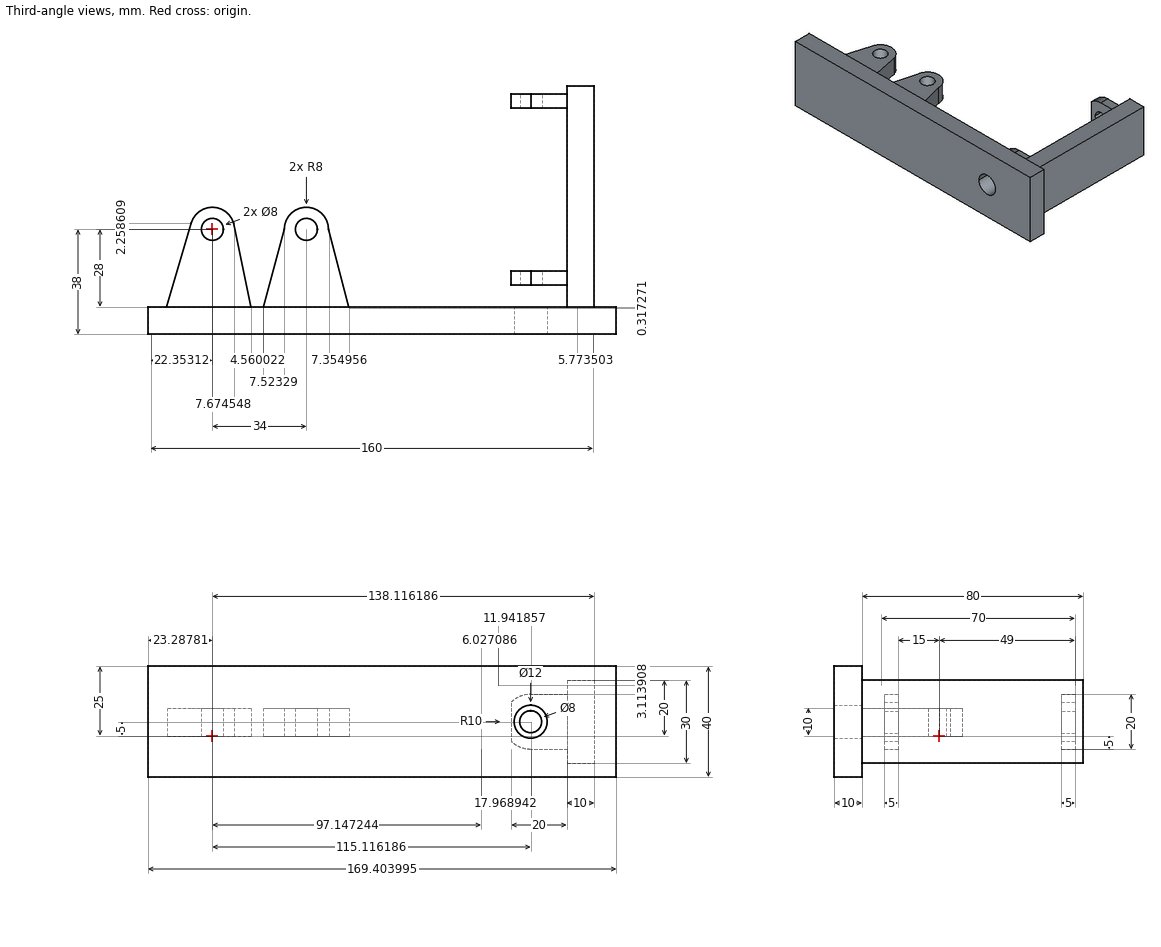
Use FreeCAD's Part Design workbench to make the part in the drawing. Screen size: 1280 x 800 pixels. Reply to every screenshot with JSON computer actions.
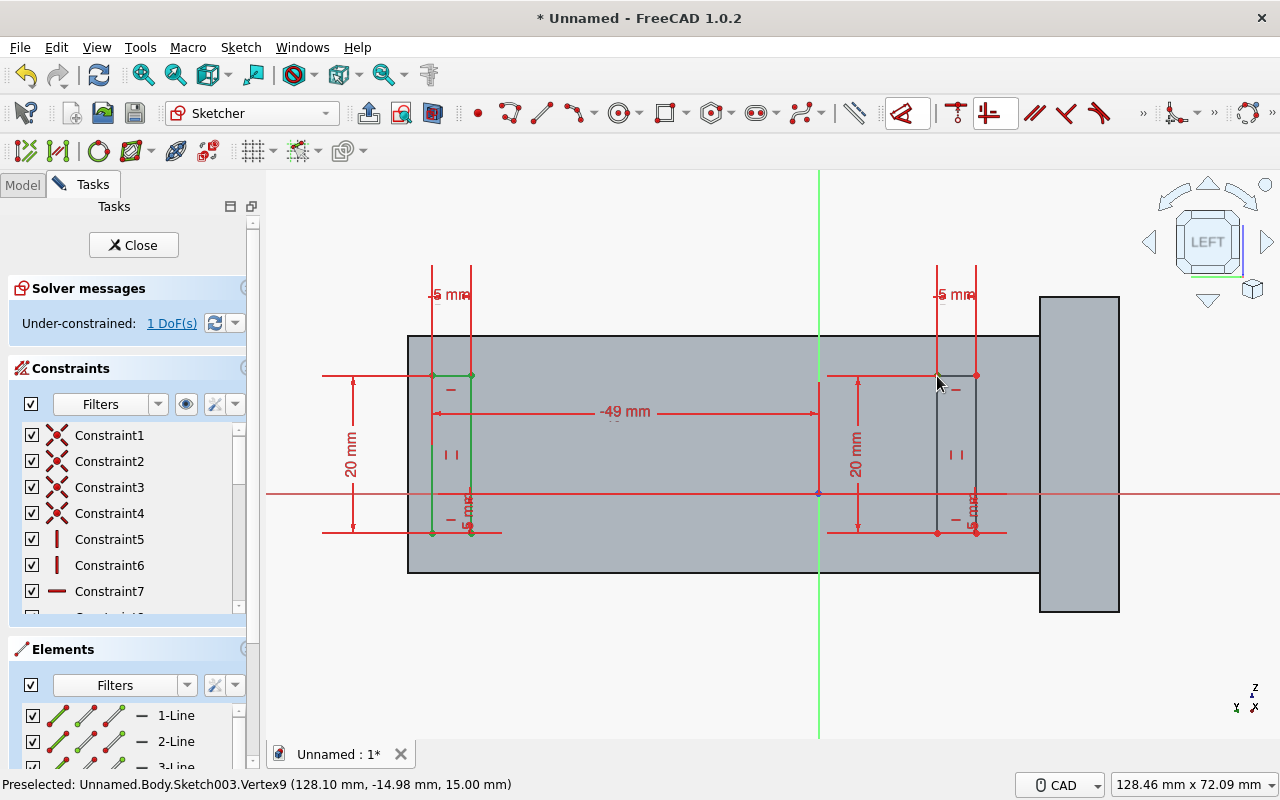
{"action": "key", "text": "l"}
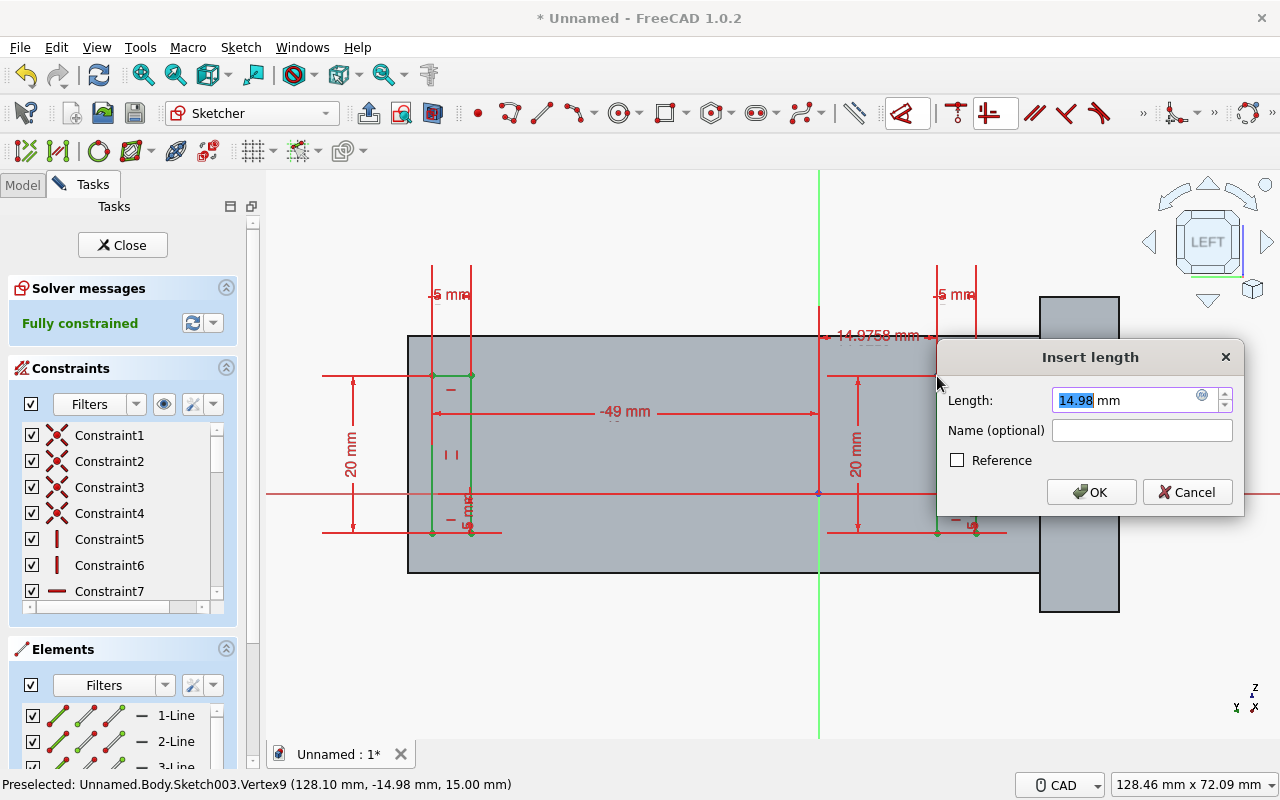
{"action": "type", "text": "15"}
{"action": "key", "text": "Return"}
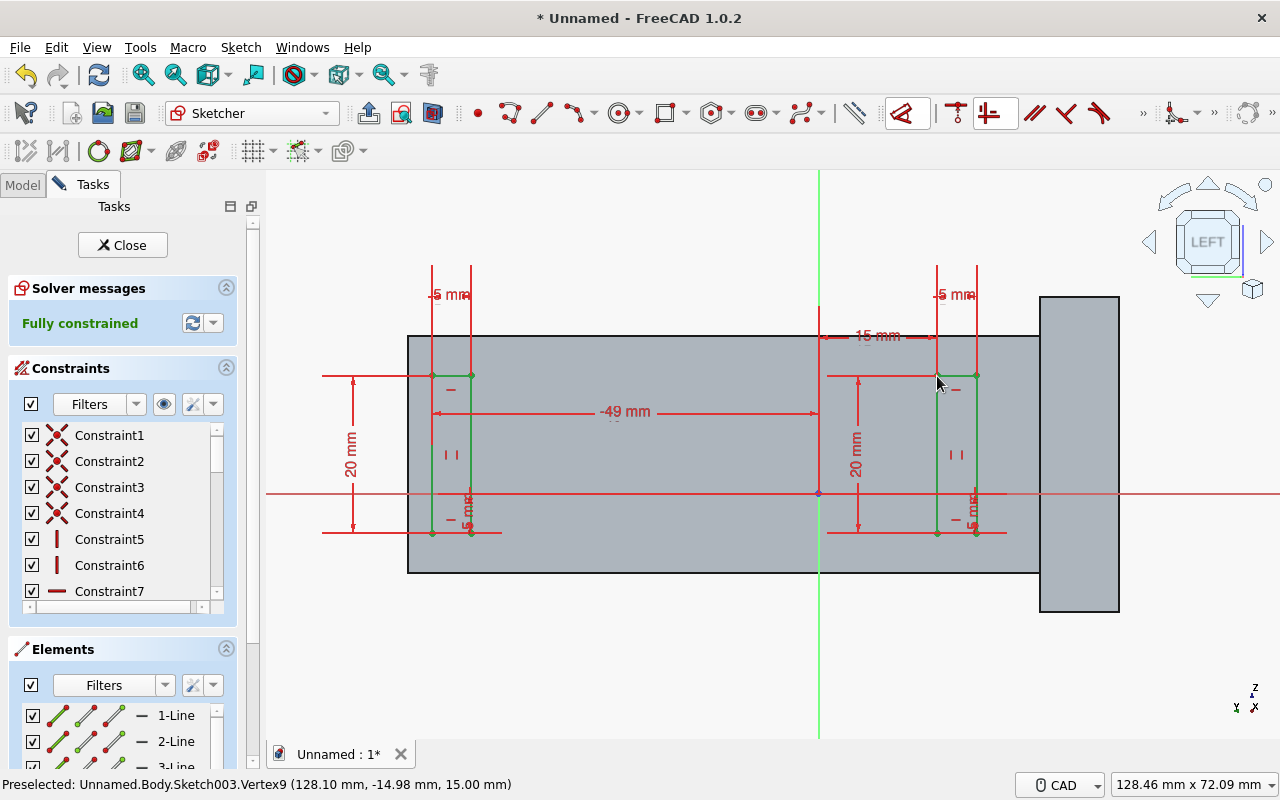
{"action": "left_click", "coordinate": [123, 245]}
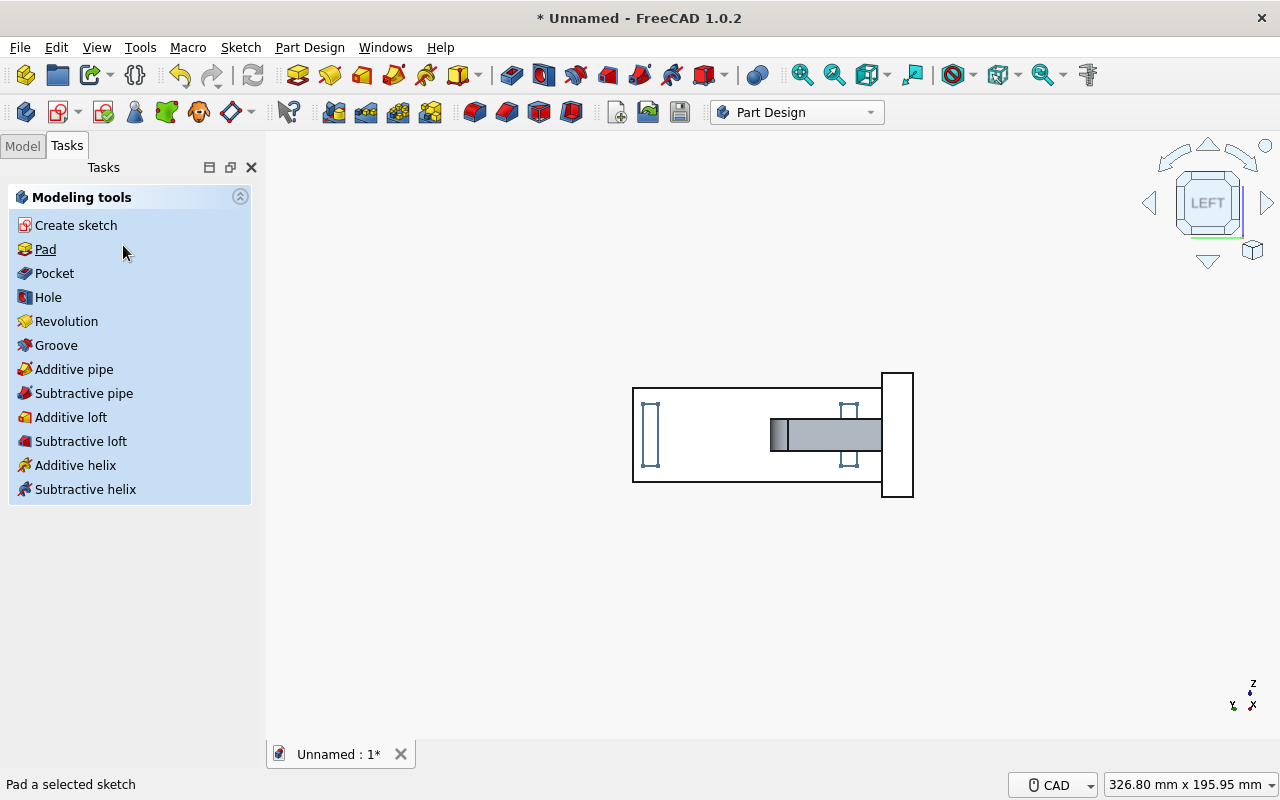
{"action": "left_click", "coordinate": [298, 76]}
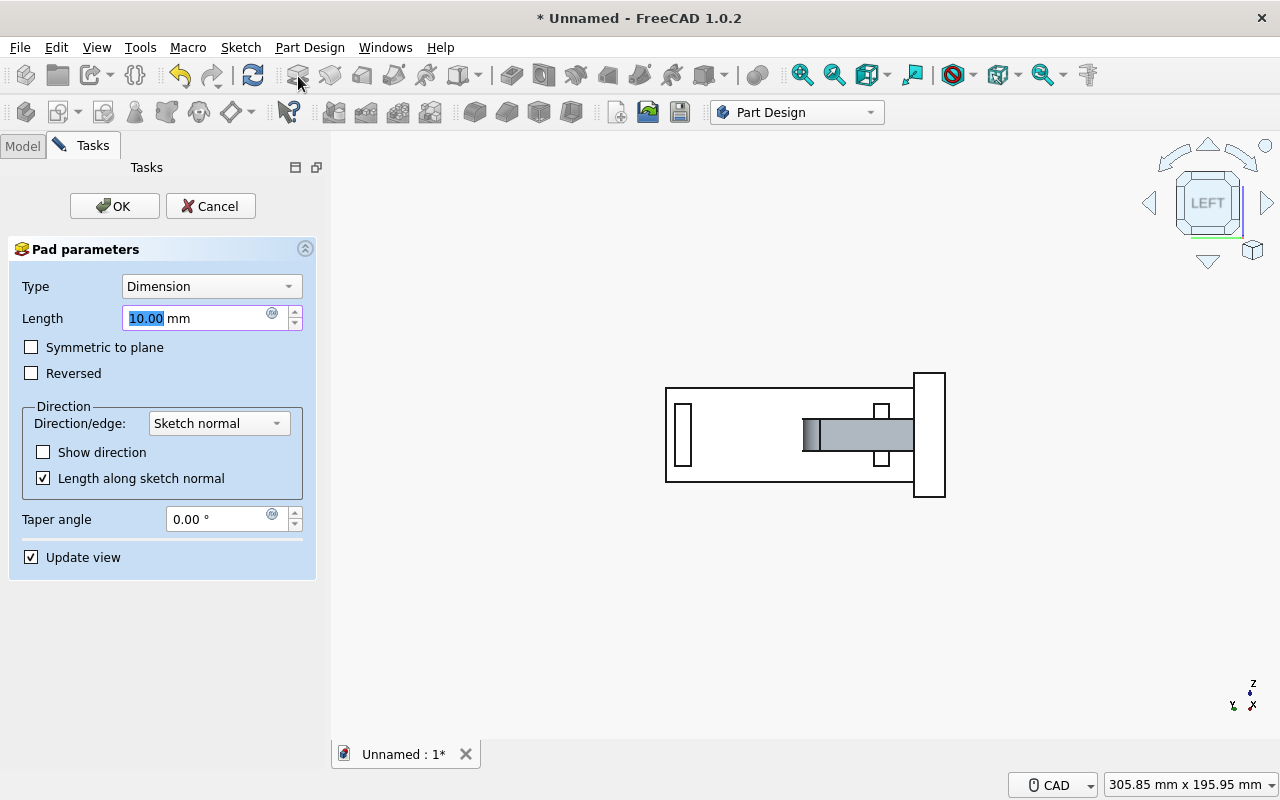
{"action": "type", "text": "20"}
{"action": "key", "text": "Tab"}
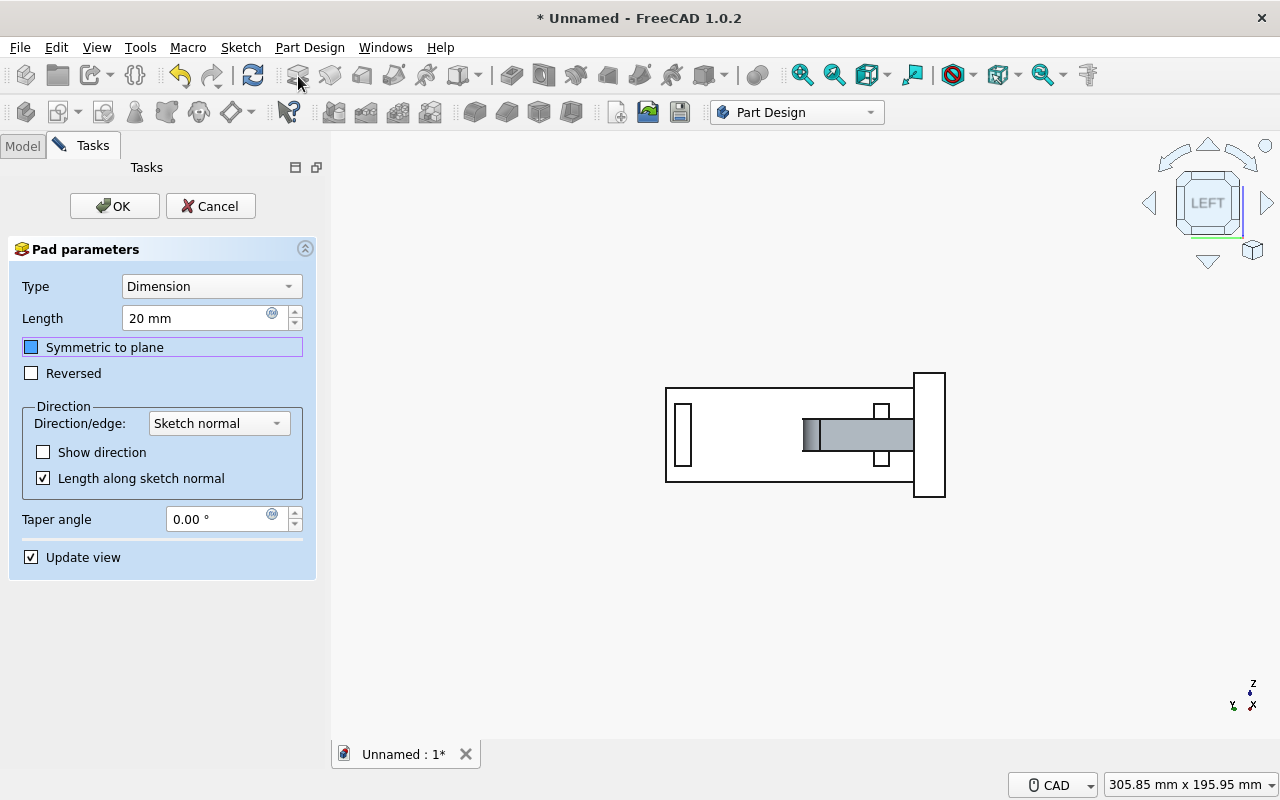
{"action": "left_click", "coordinate": [115, 206]}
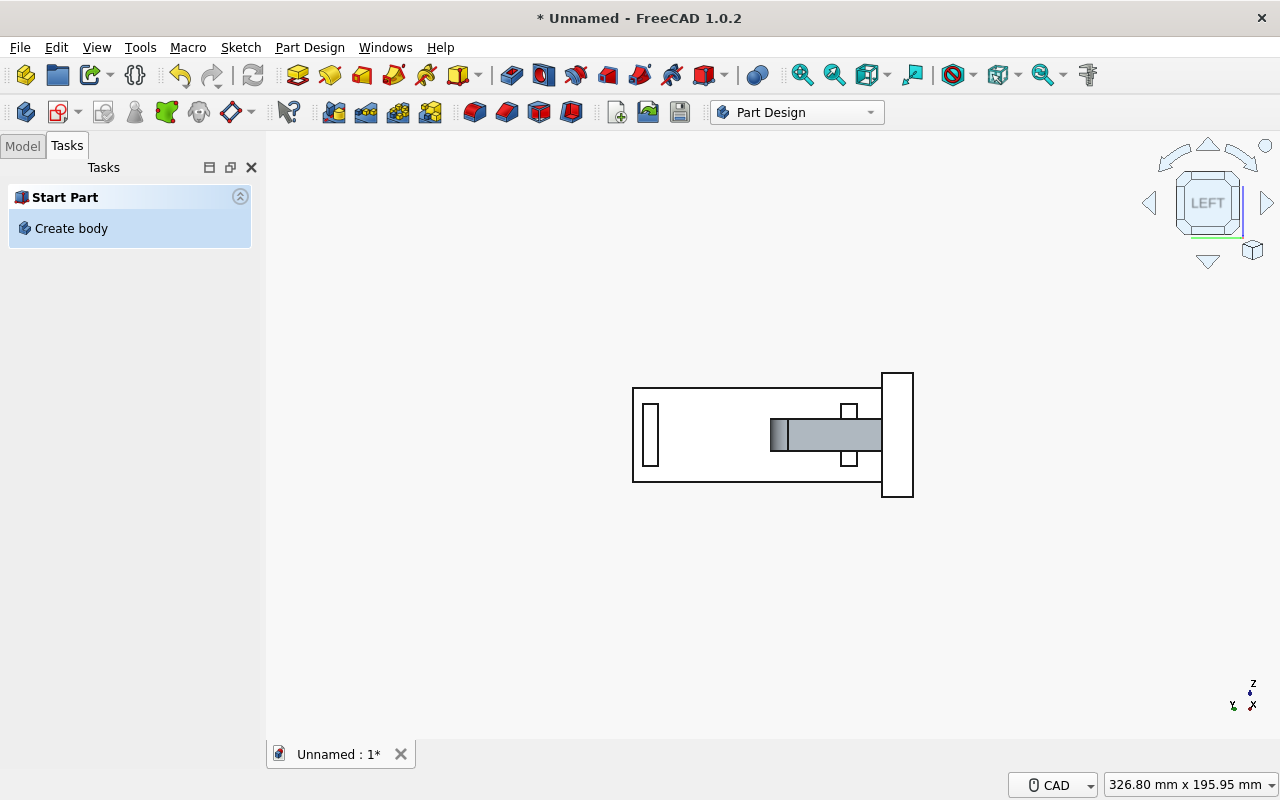
{"action": "left_click", "coordinate": [804, 76]}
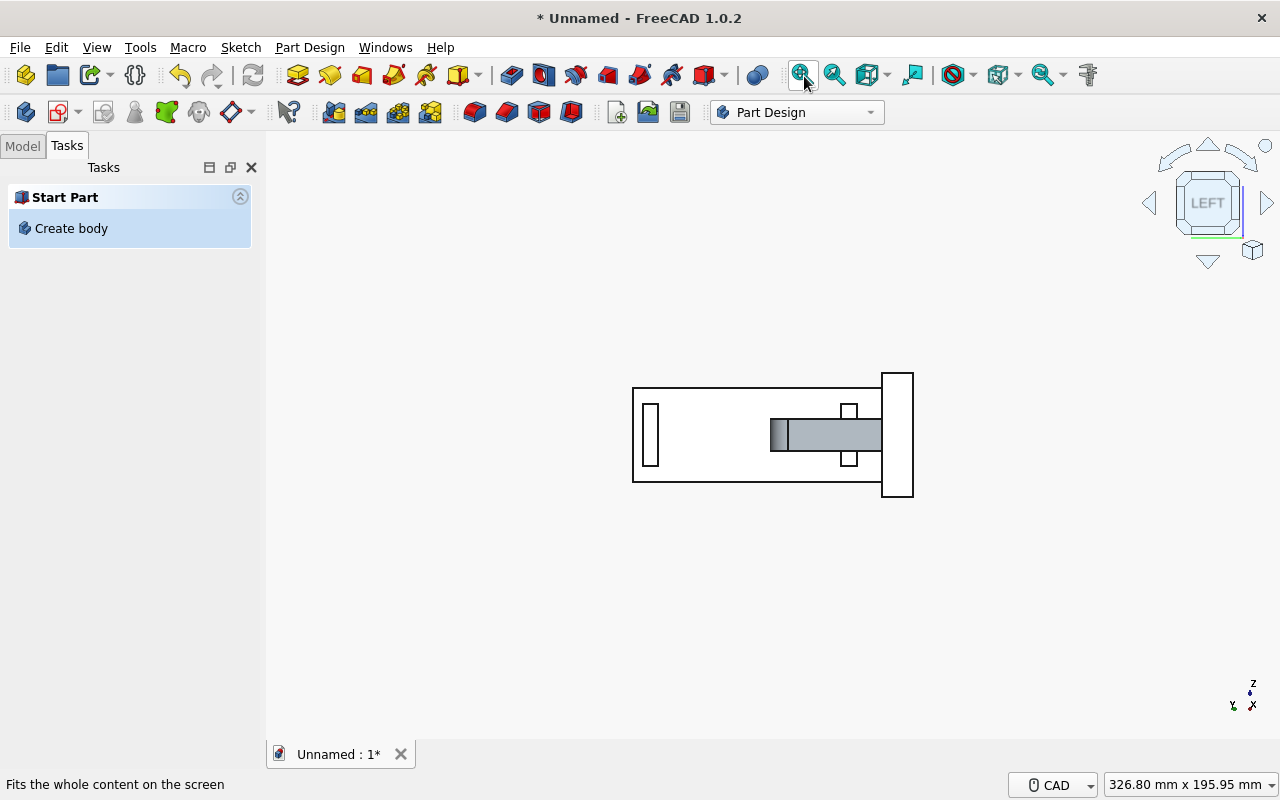
{"action": "key", "text": "4"}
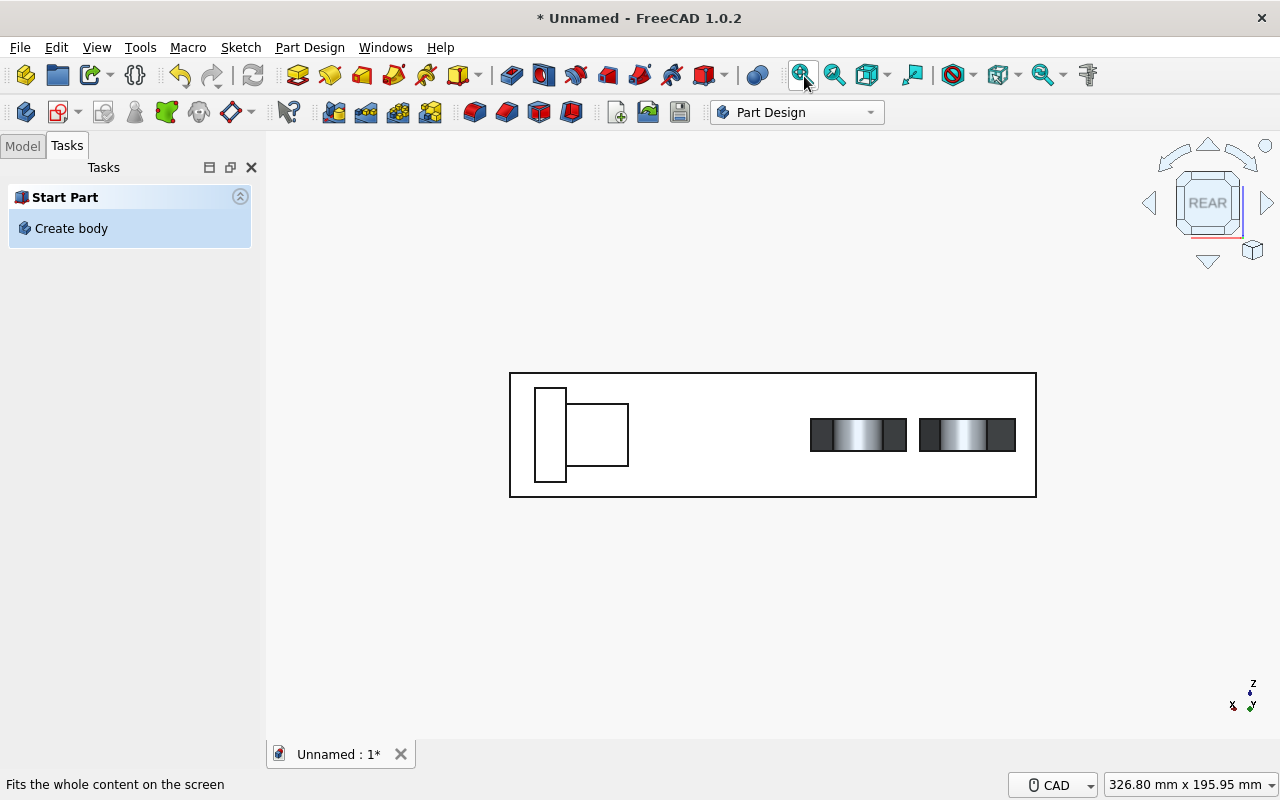
{"action": "left_click", "coordinate": [597, 434]}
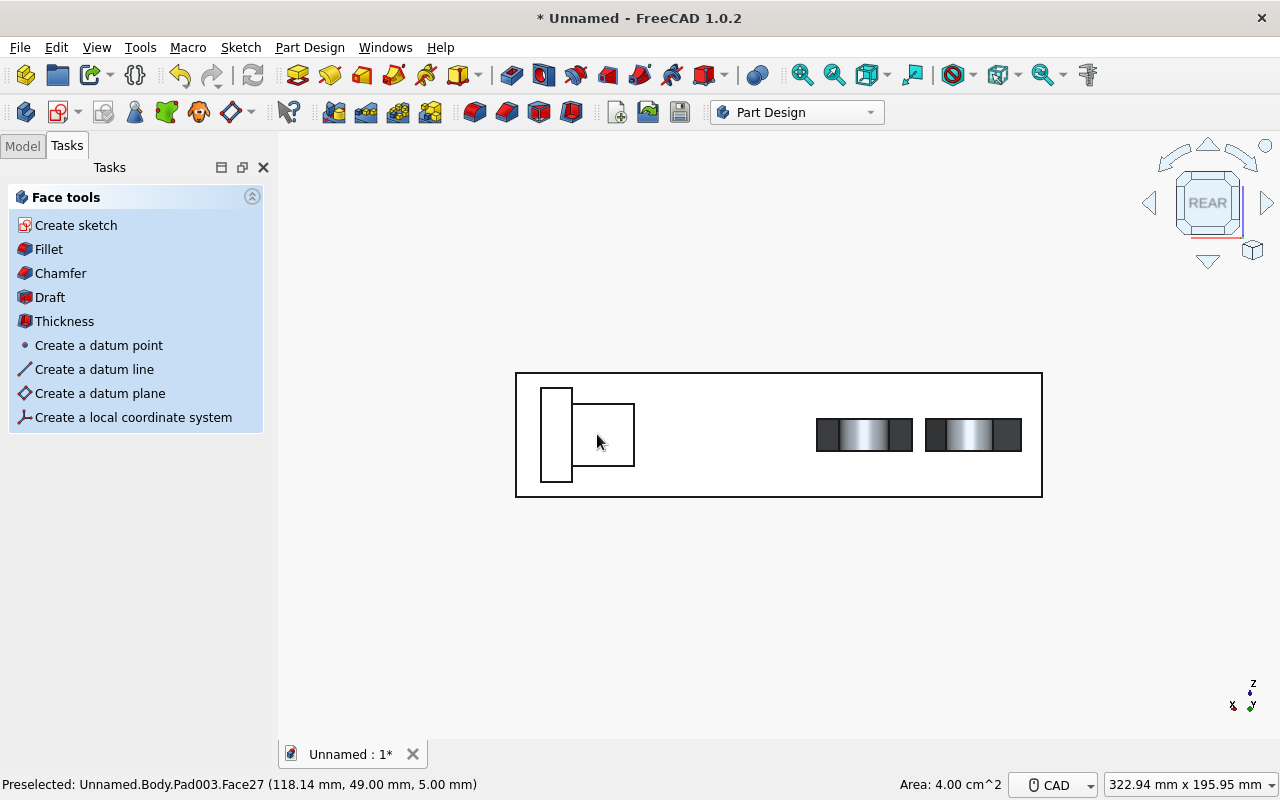
{"action": "left_click", "coordinate": [58, 112]}